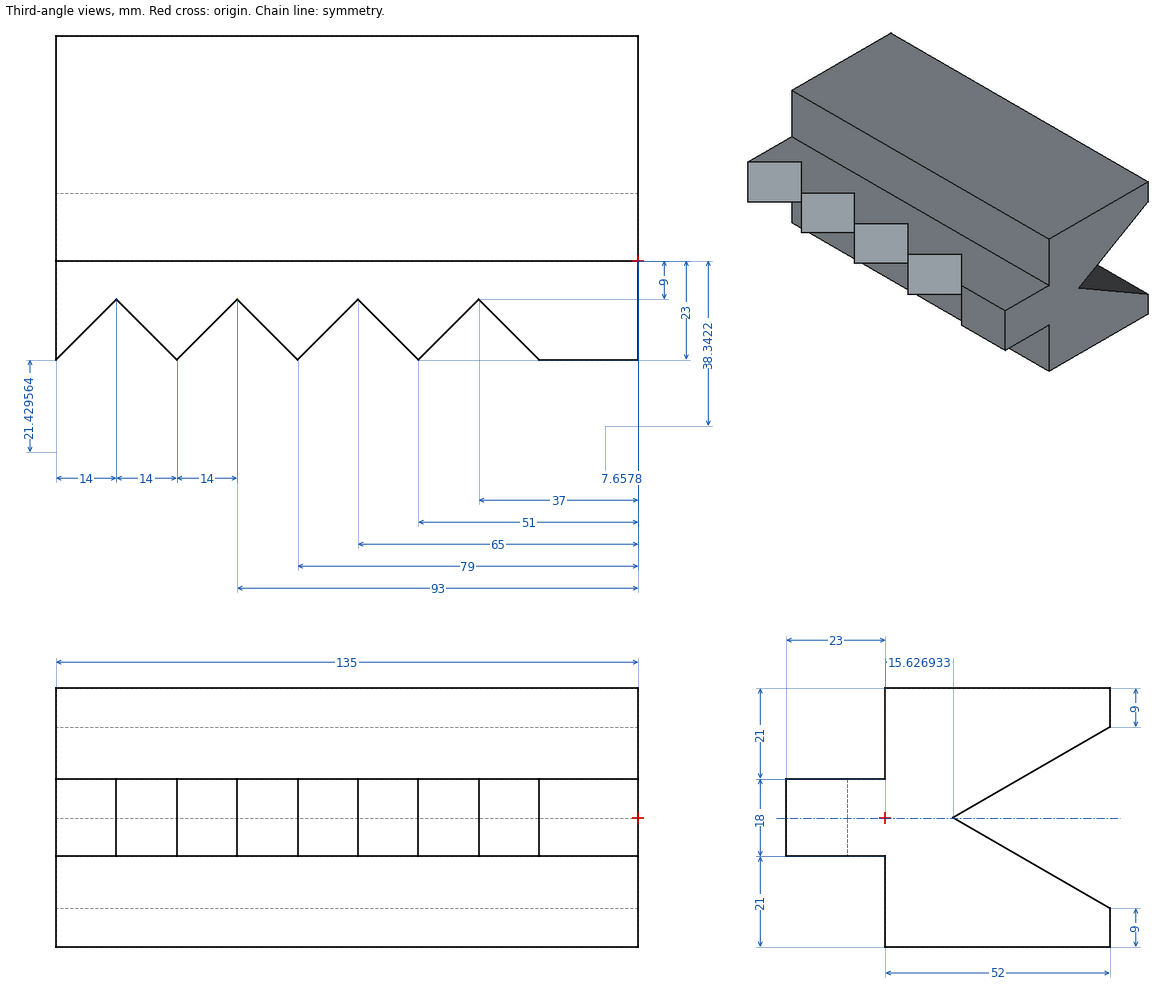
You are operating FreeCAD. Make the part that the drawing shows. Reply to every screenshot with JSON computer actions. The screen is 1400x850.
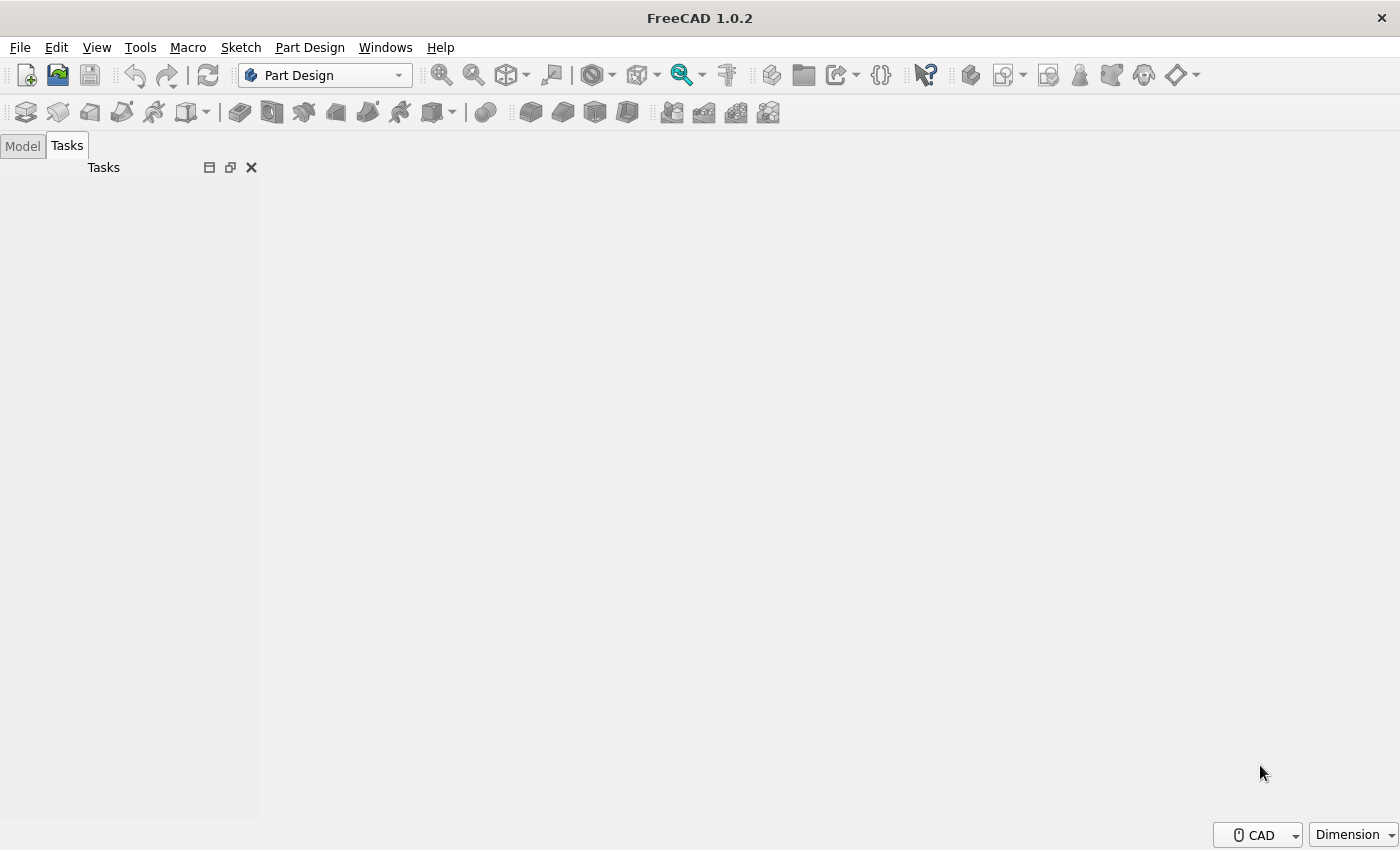
{"action": "left_click", "coordinate": [26, 76]}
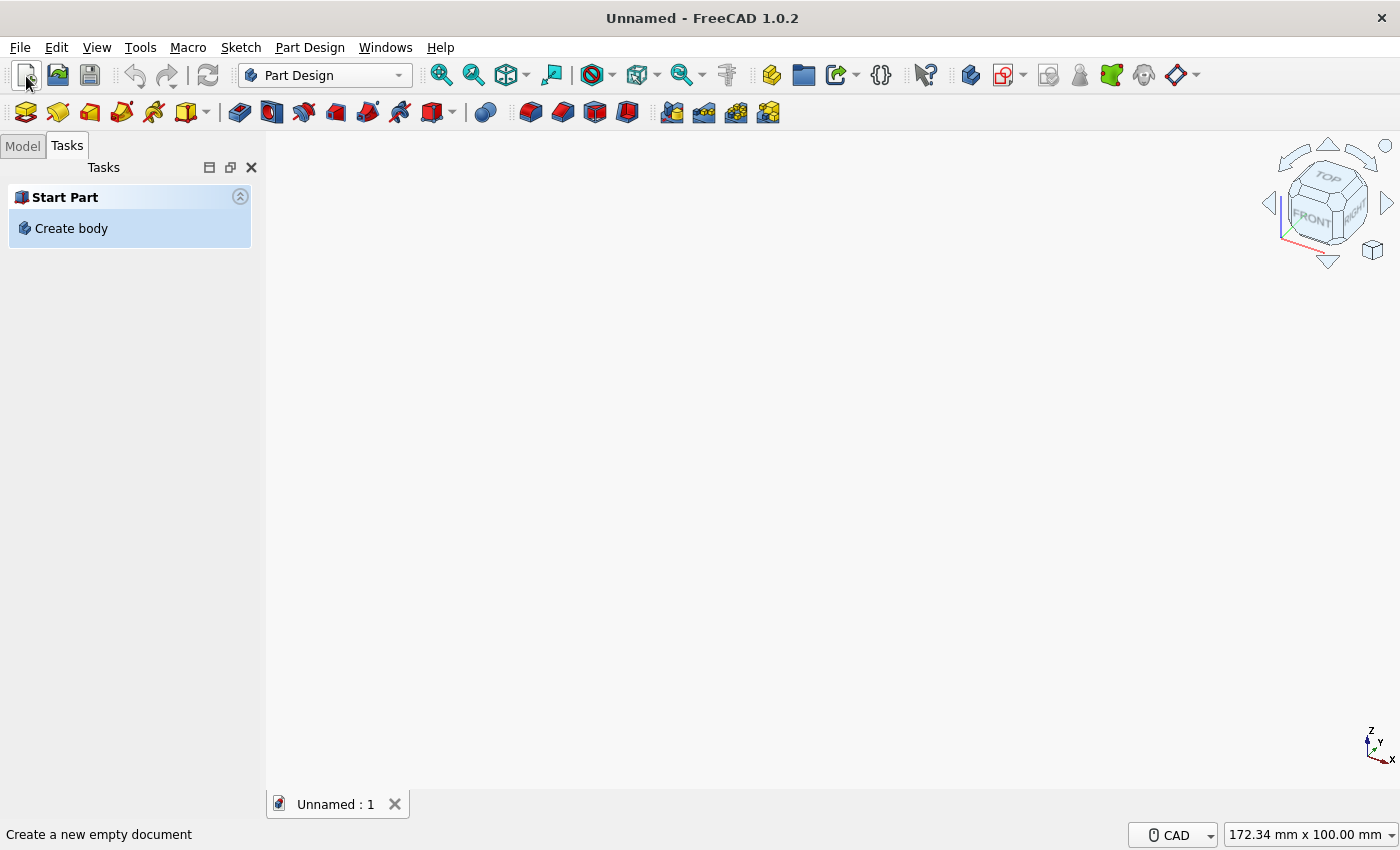
{"action": "left_click", "coordinate": [1004, 76]}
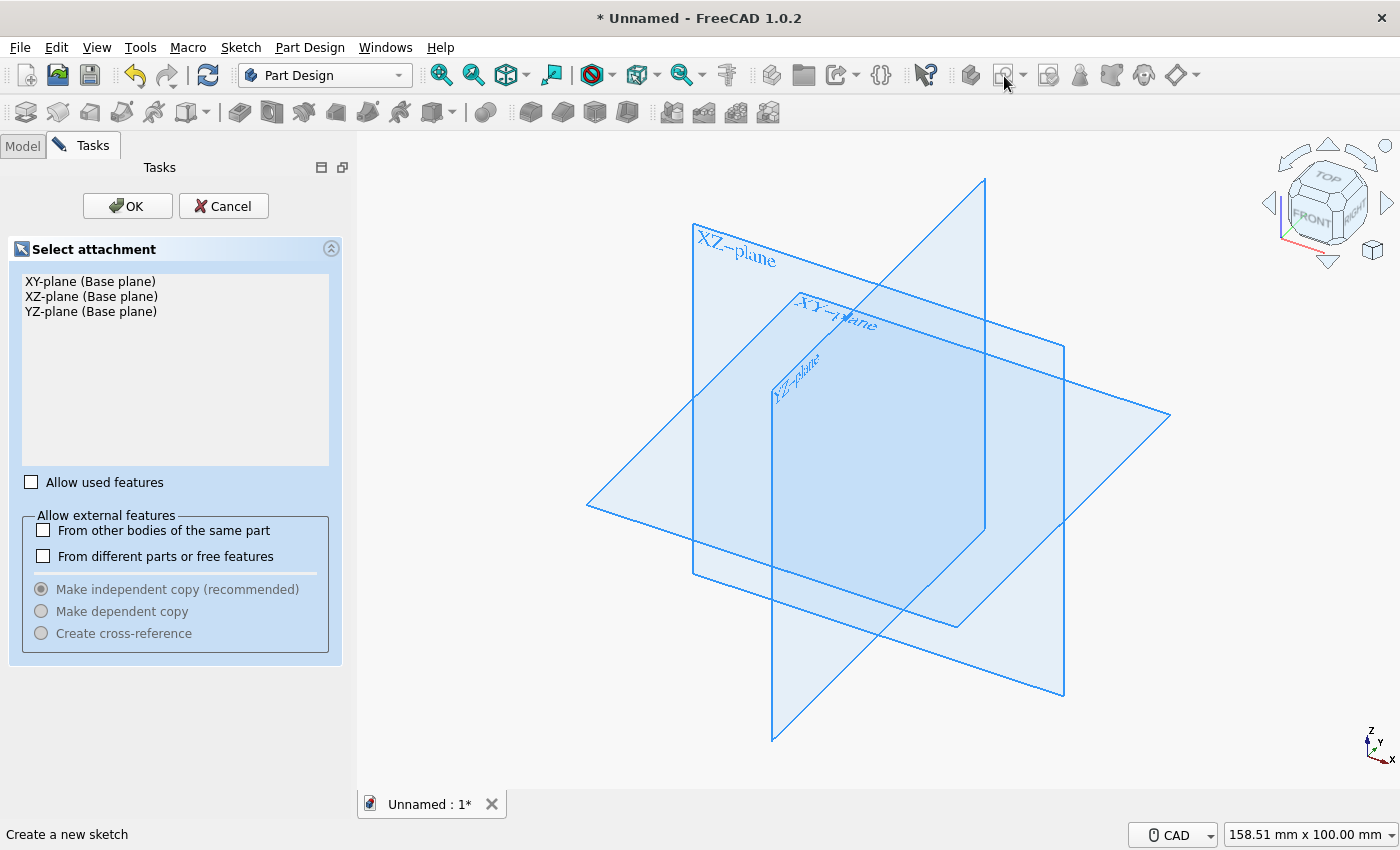
{"action": "left_click", "coordinate": [82, 312]}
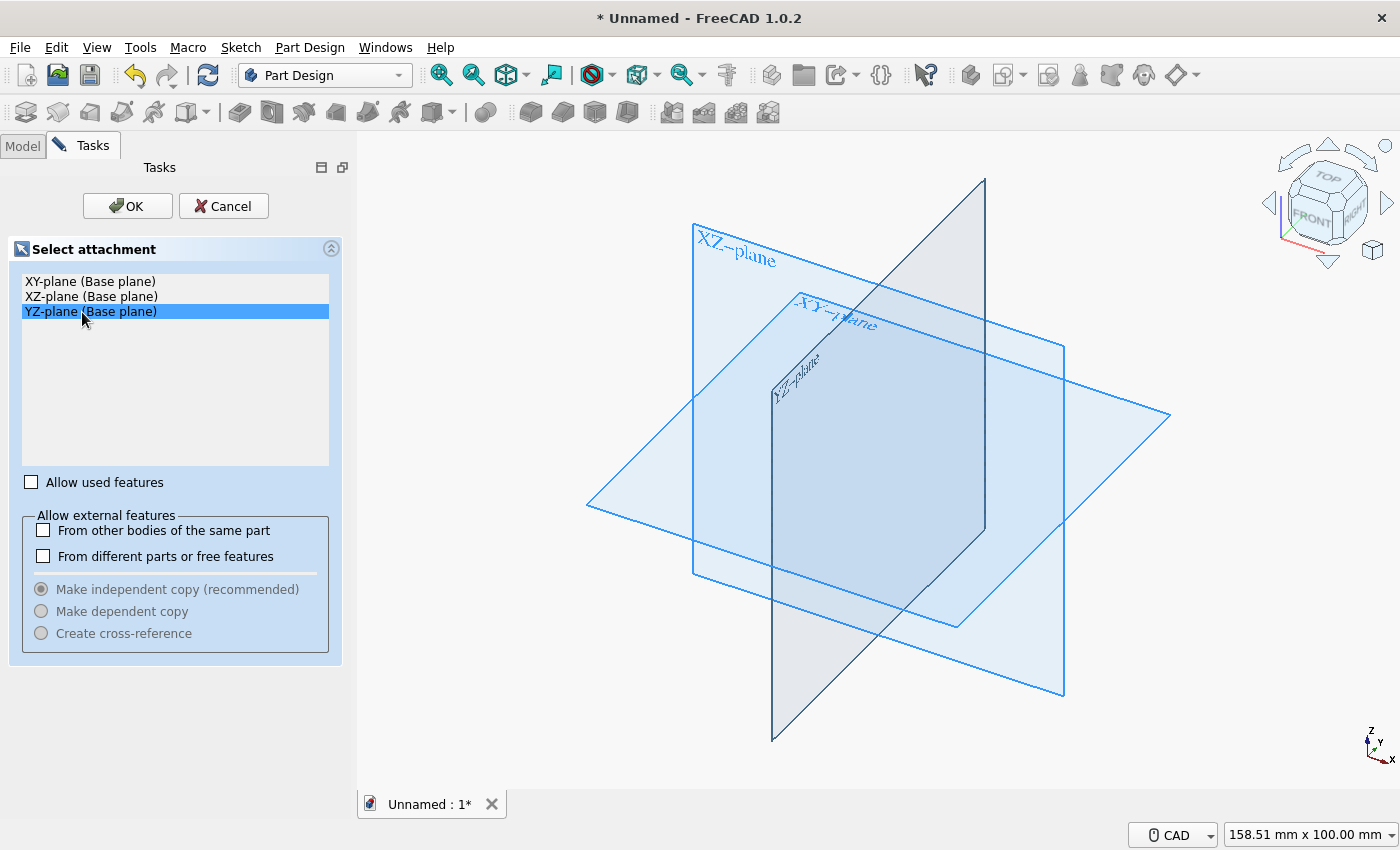
{"action": "left_click", "coordinate": [128, 206]}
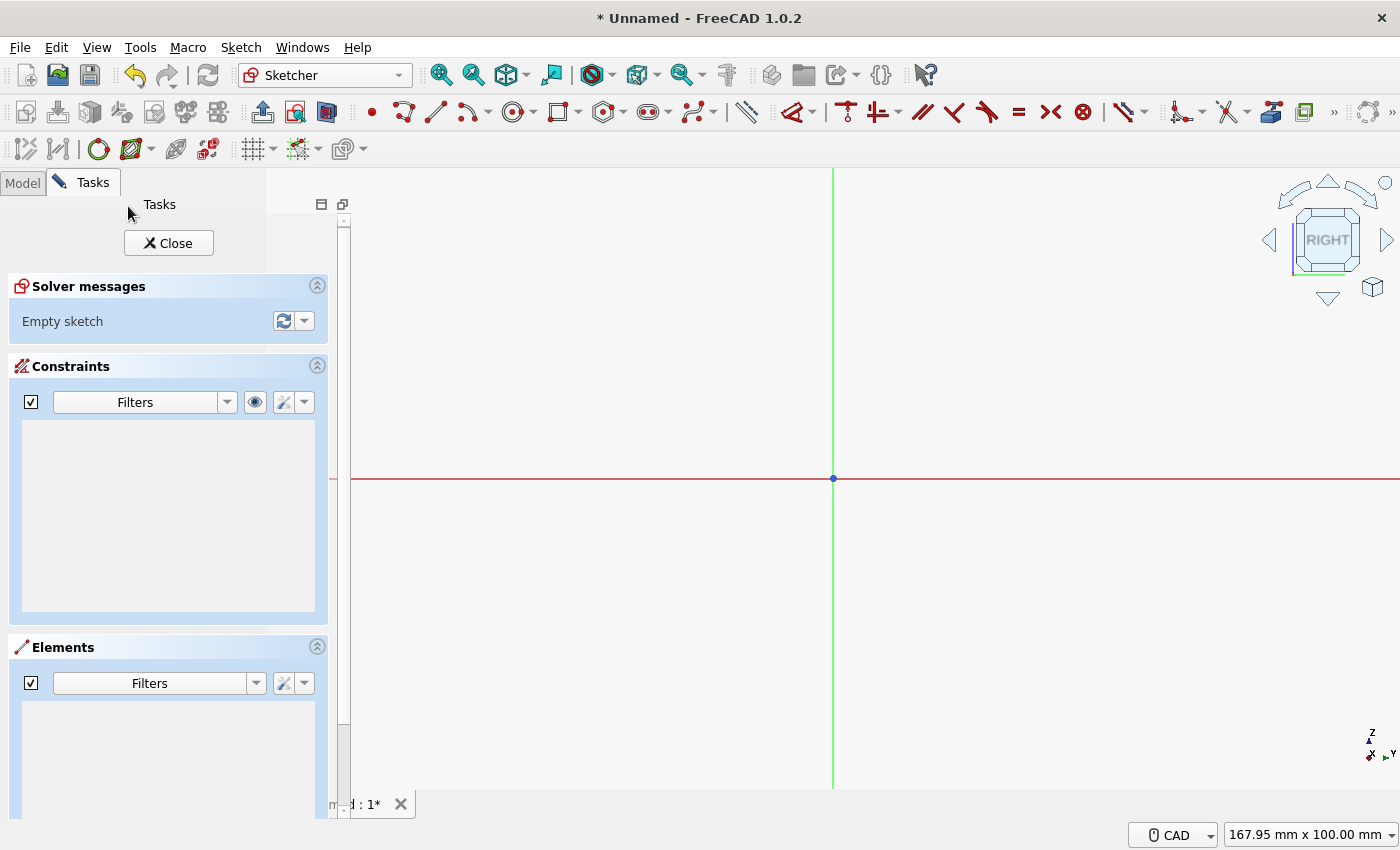
{"action": "left_click", "coordinate": [404, 112]}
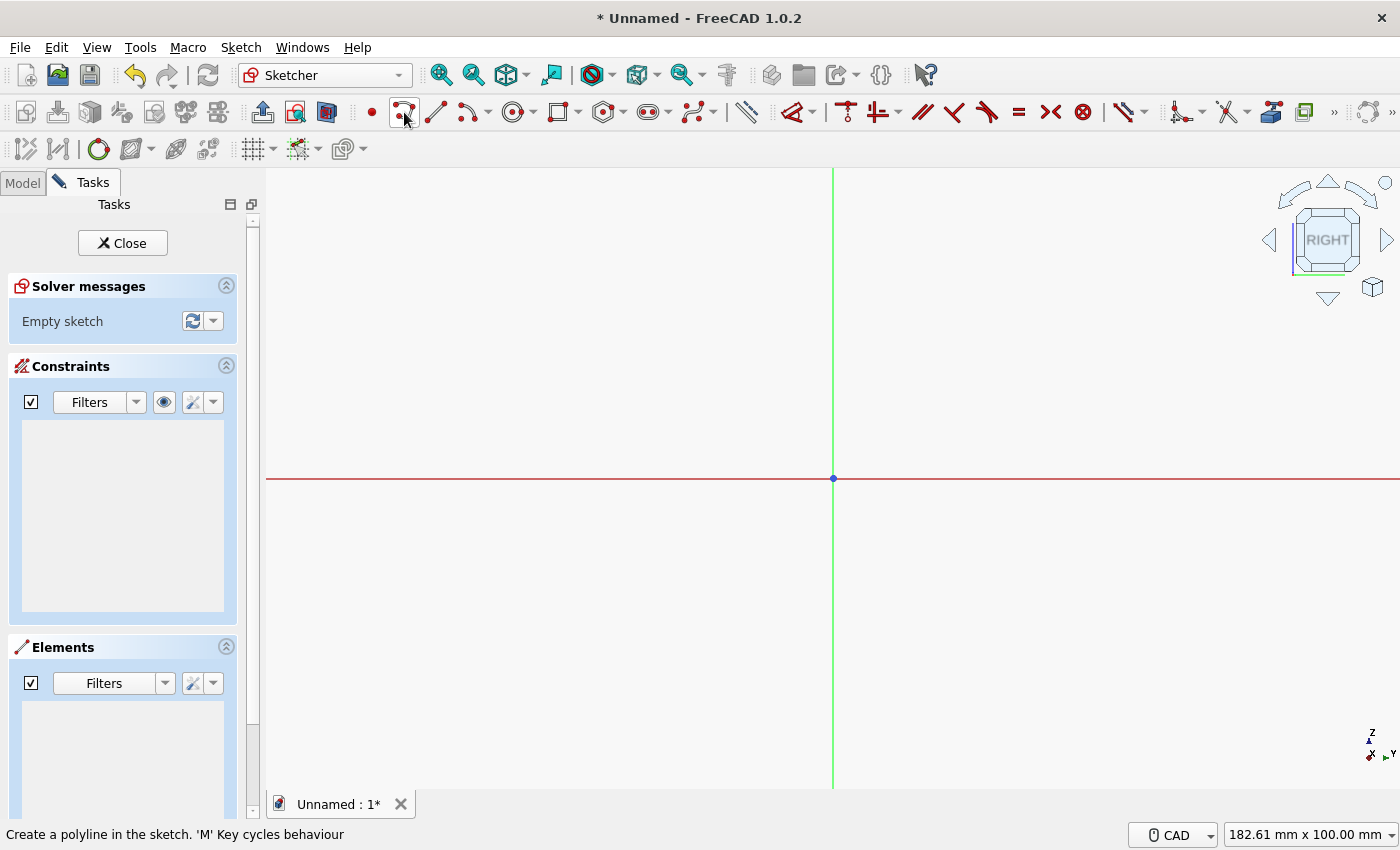
{"action": "left_click", "coordinate": [833, 423]}
{"action": "left_click", "coordinate": [690, 423]}
{"action": "left_click", "coordinate": [690, 534]}
{"action": "left_click", "coordinate": [833, 534]}
{"action": "left_click", "coordinate": [842, 665]}
{"action": "left_click", "coordinate": [1156, 665]}
{"action": "left_click", "coordinate": [1156, 609]}
{"action": "left_click", "coordinate": [930, 478]}
{"action": "left_click", "coordinate": [1156, 348]}
{"action": "left_click", "coordinate": [1156, 292]}
{"action": "left_click", "coordinate": [842, 292]}
{"action": "left_click", "coordinate": [833, 424]}
{"action": "key", "text": "Escape"}
{"action": "key", "text": "Escape"}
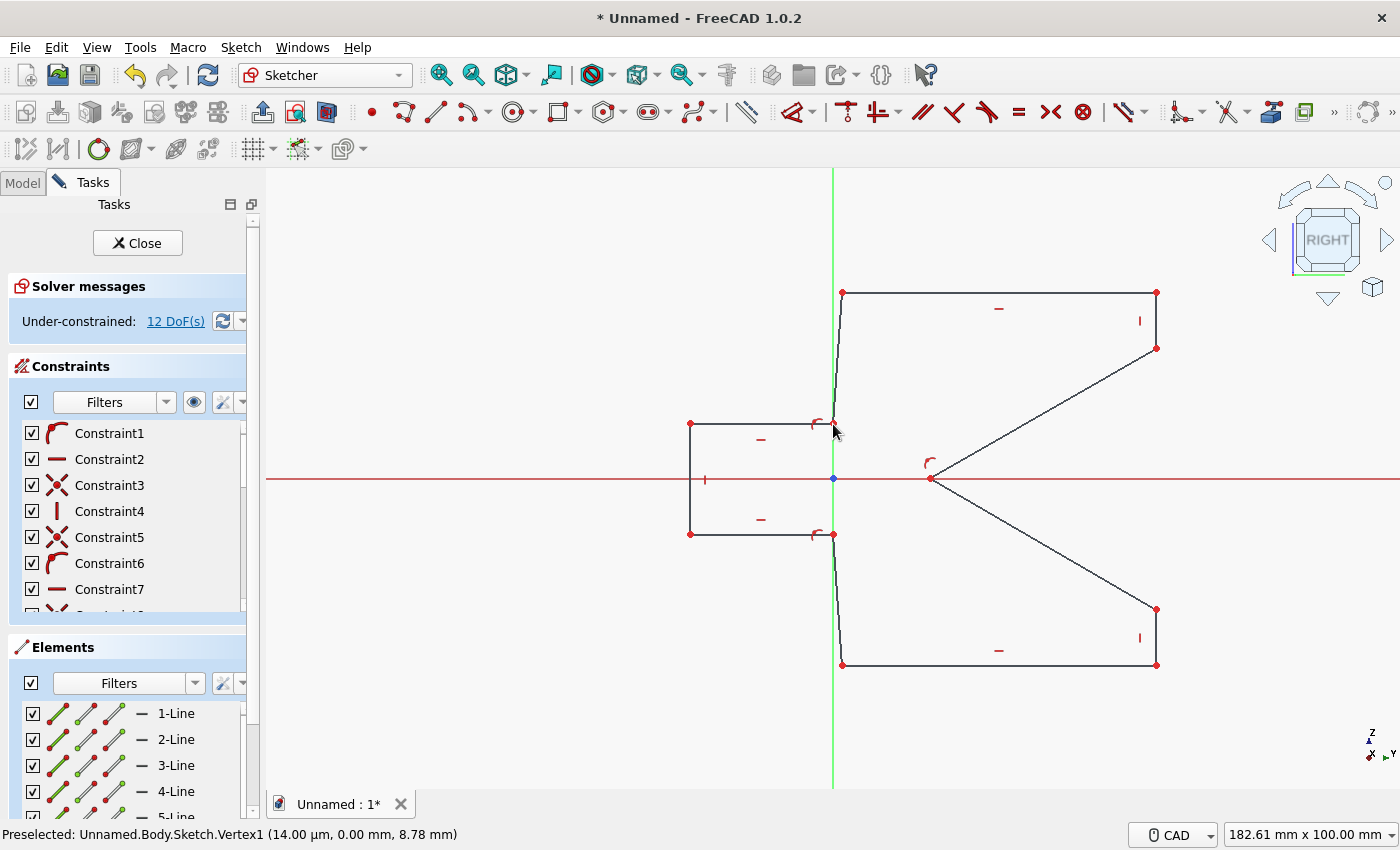
{"action": "left_click", "coordinate": [836, 574]}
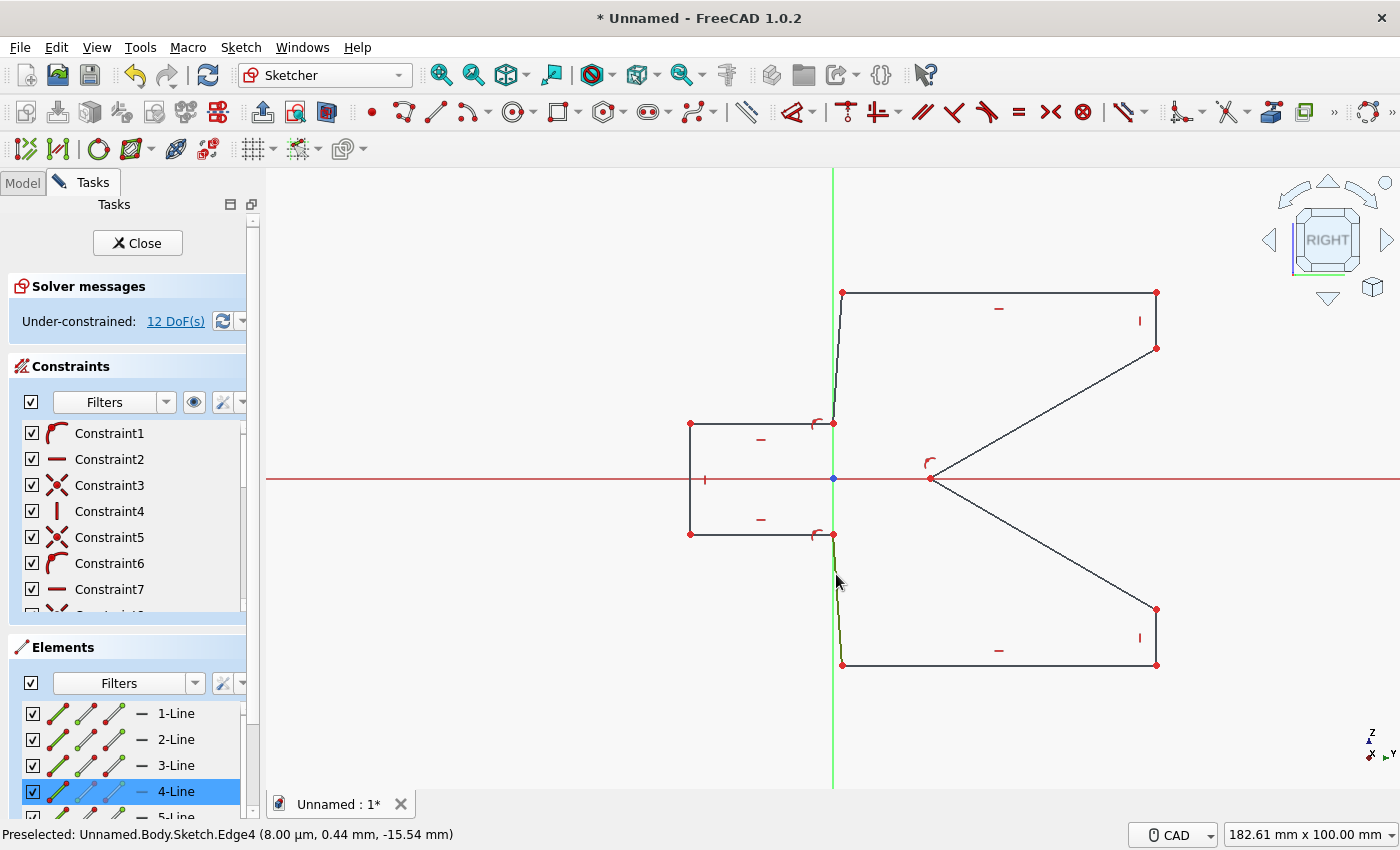
{"action": "left_click", "coordinate": [900, 112]}